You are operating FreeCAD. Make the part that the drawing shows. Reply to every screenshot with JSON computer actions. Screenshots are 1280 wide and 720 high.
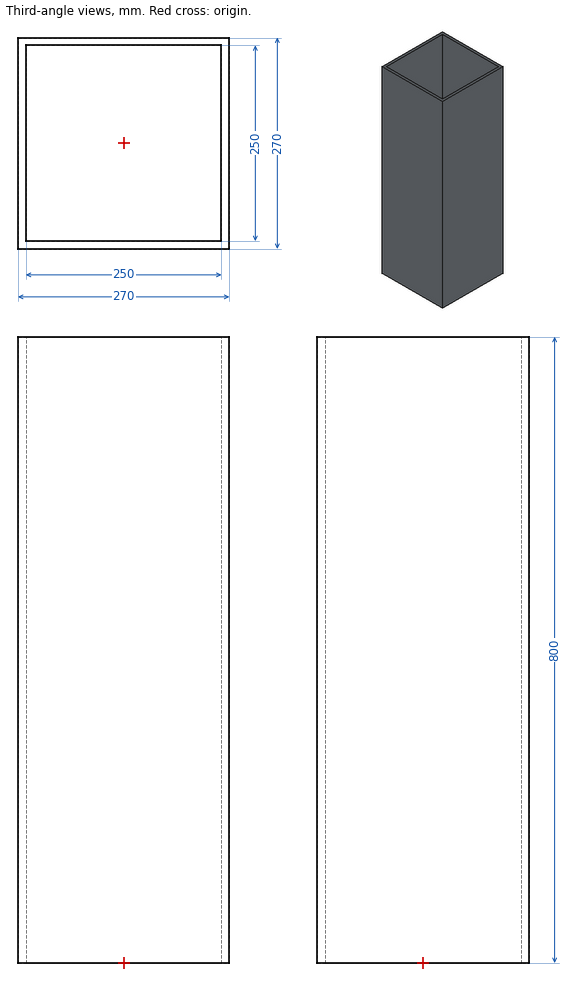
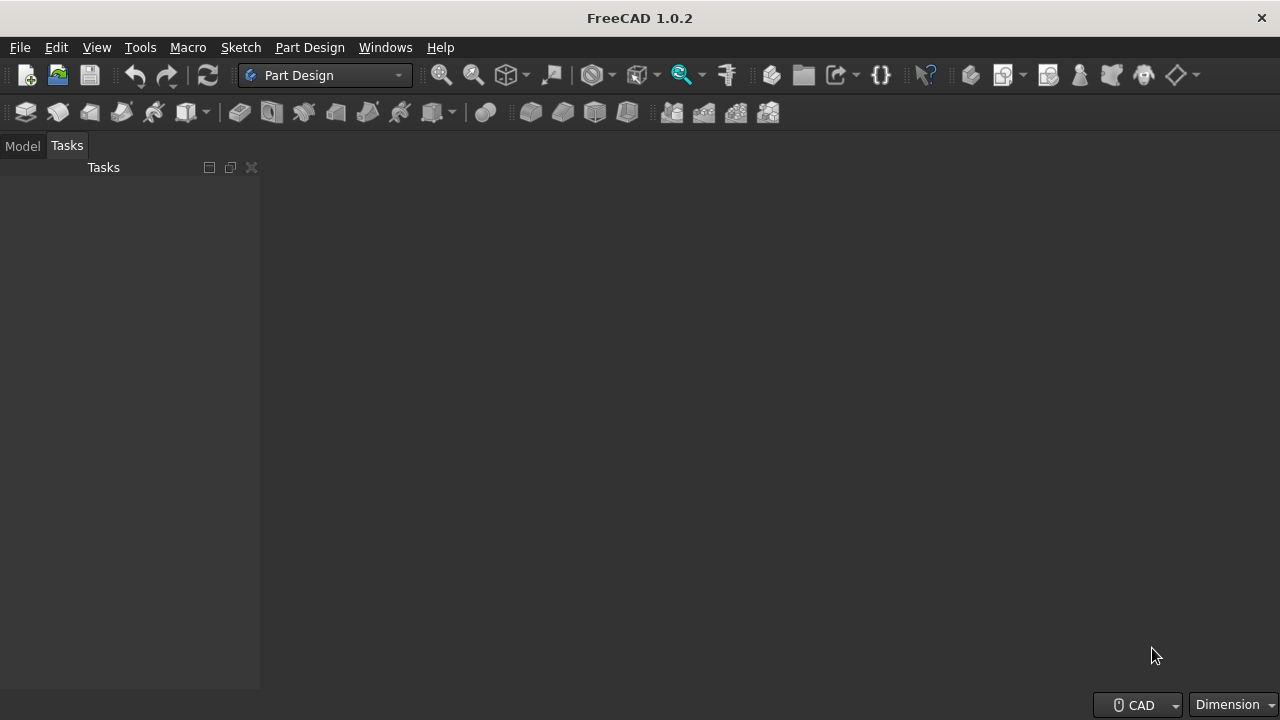
{"action": "left_click", "coordinate": [26, 76]}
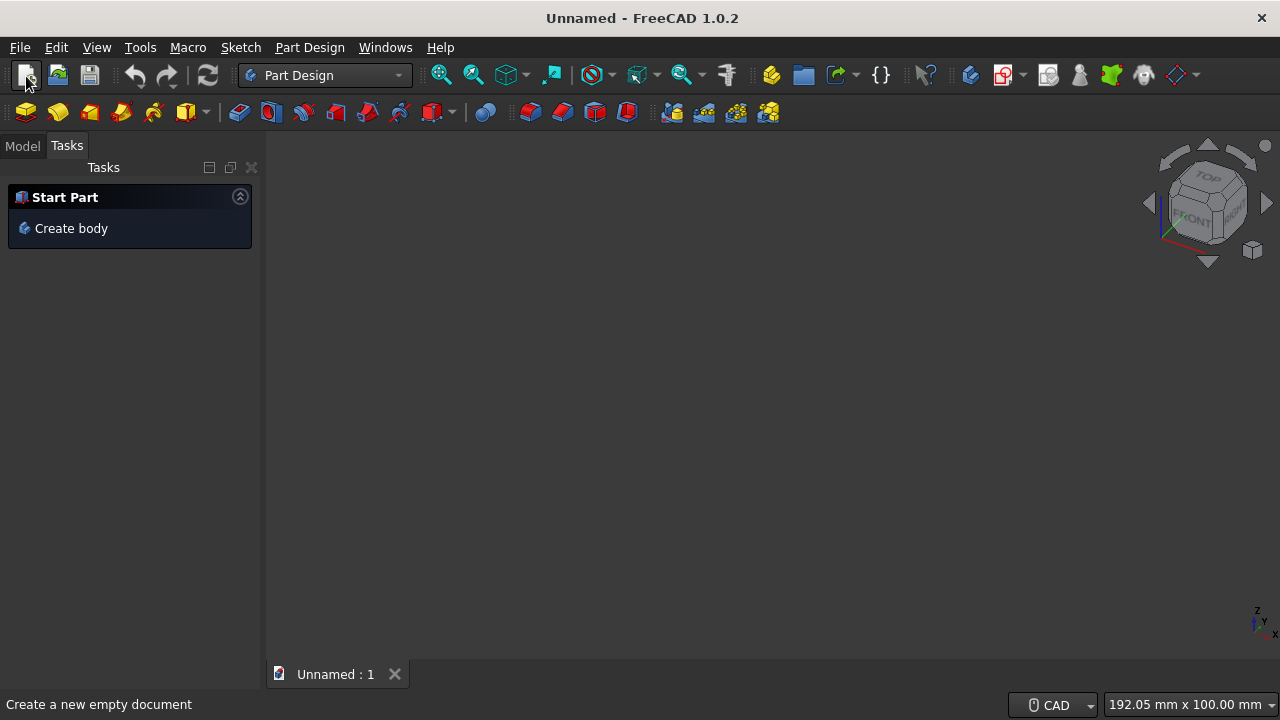
{"action": "left_click", "coordinate": [1004, 76]}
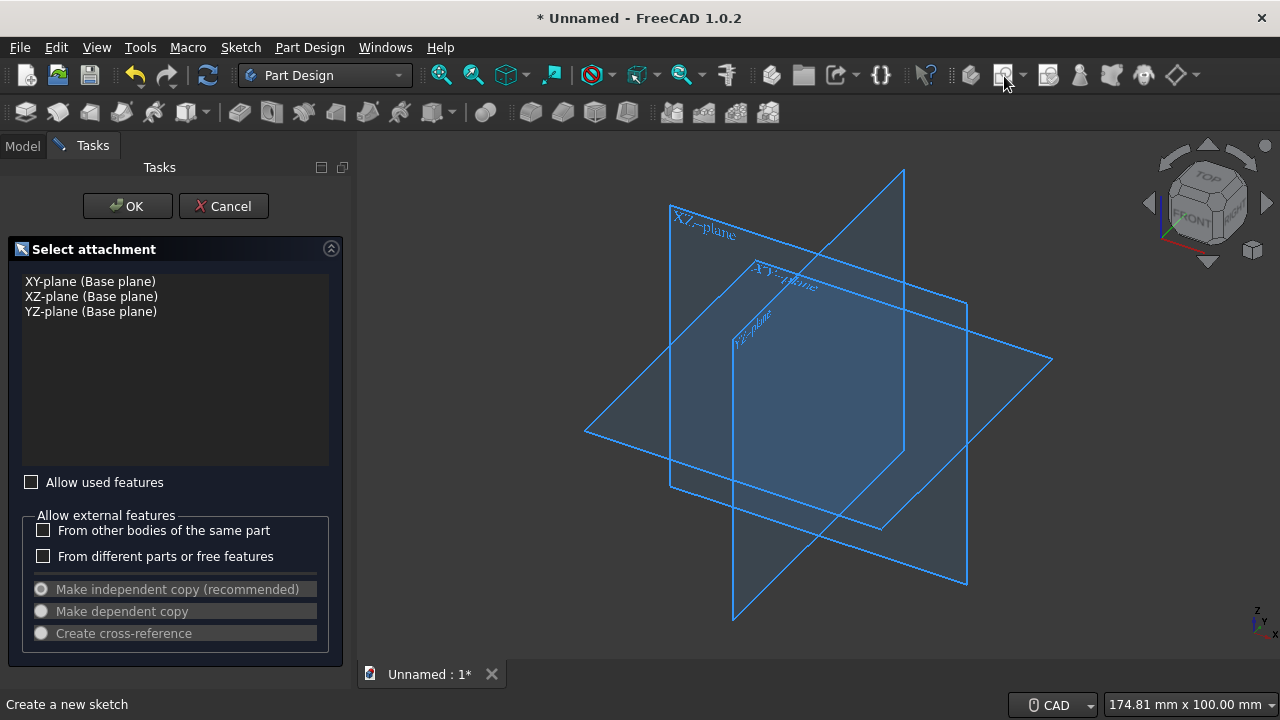
{"action": "left_click", "coordinate": [82, 282]}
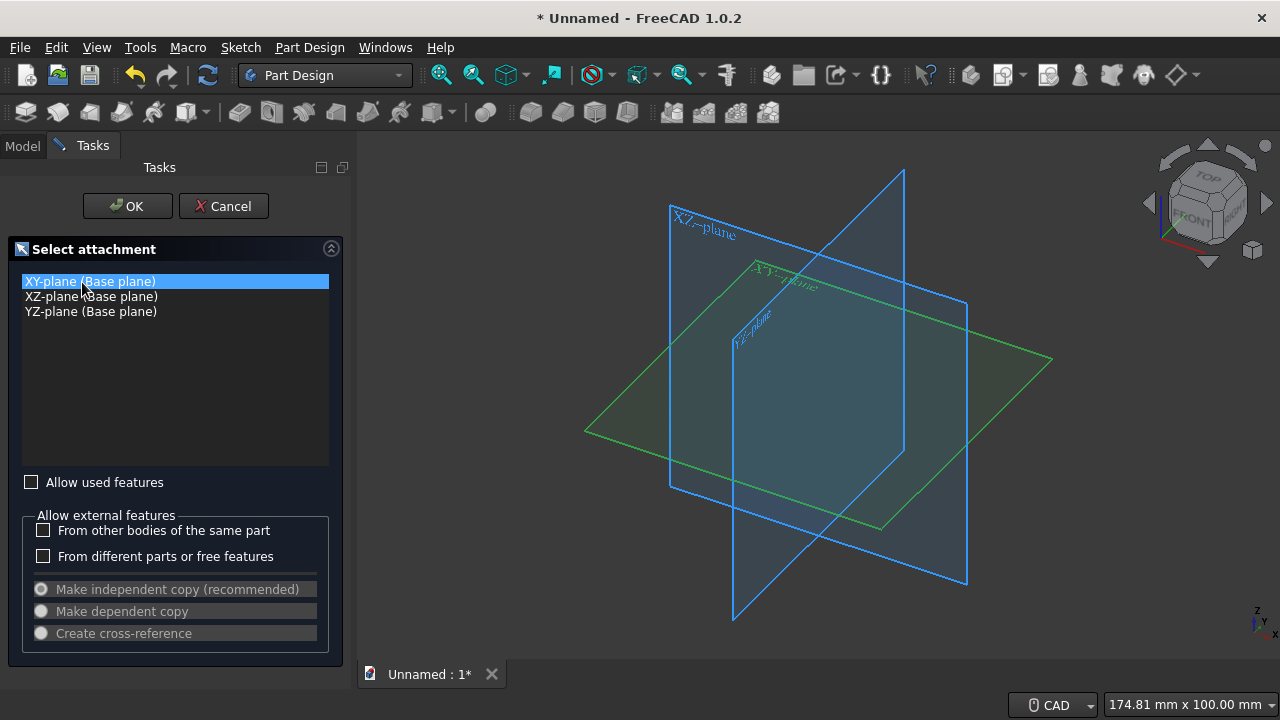
{"action": "left_click", "coordinate": [128, 206]}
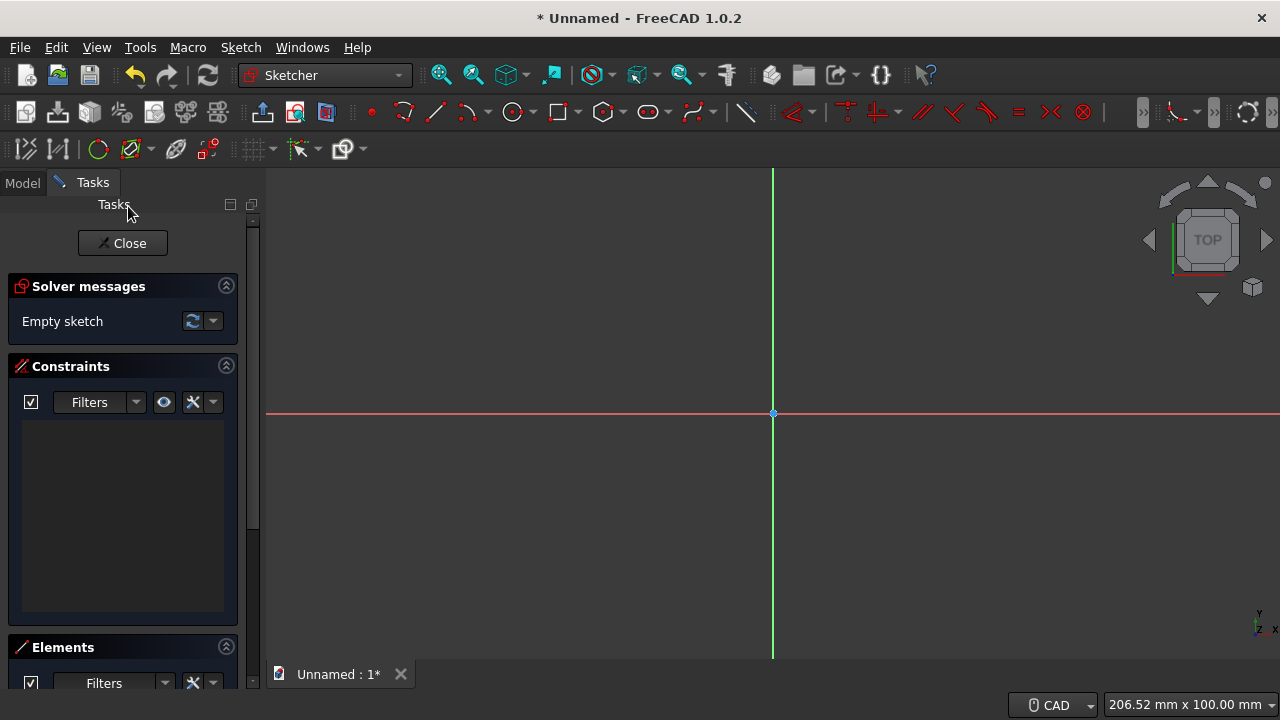
{"action": "scroll", "coordinate": [682, 414], "scroll_direction": "down", "scroll_amount": 7}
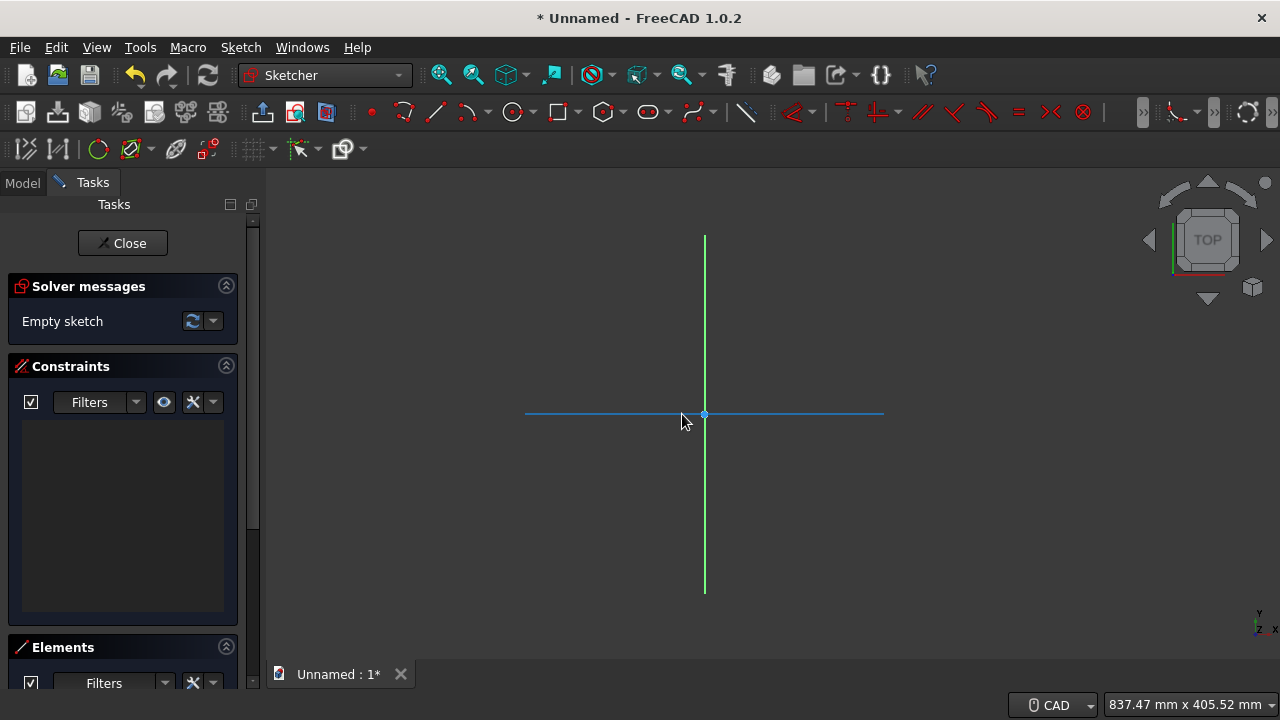
{"action": "key", "text": "g v"}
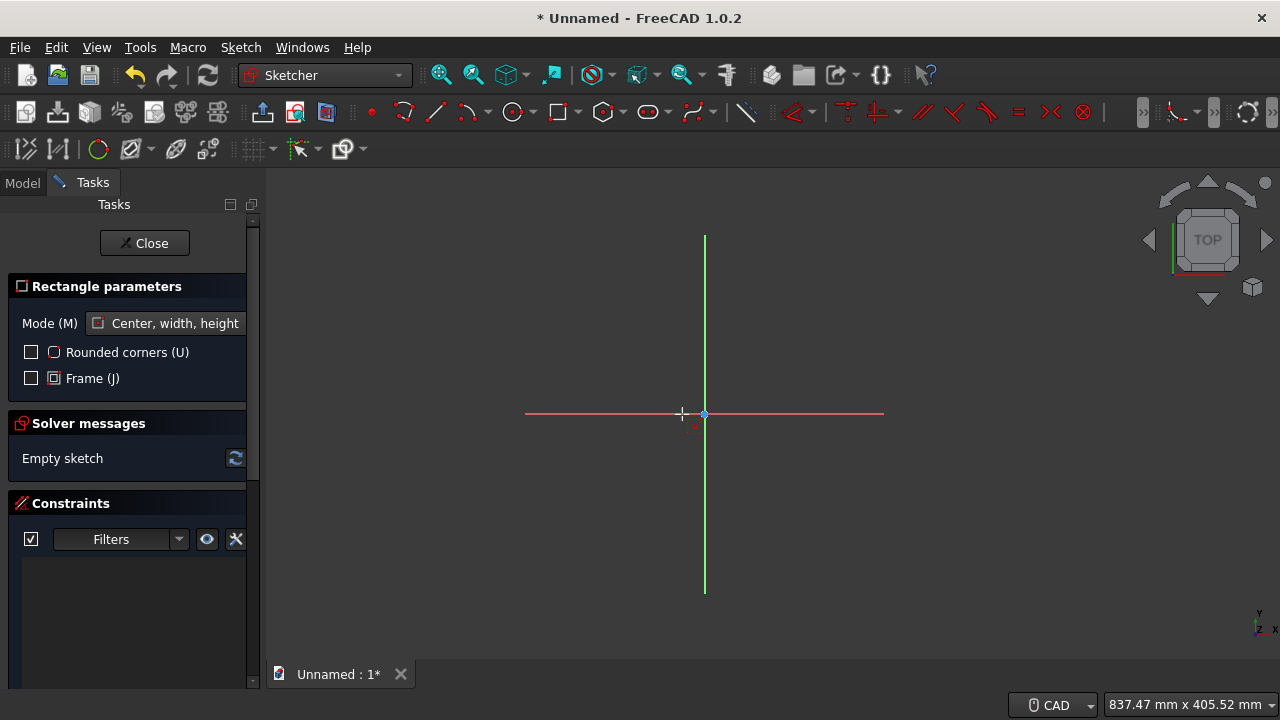
{"action": "left_click", "coordinate": [705, 414]}
{"action": "left_click", "coordinate": [868, 251]}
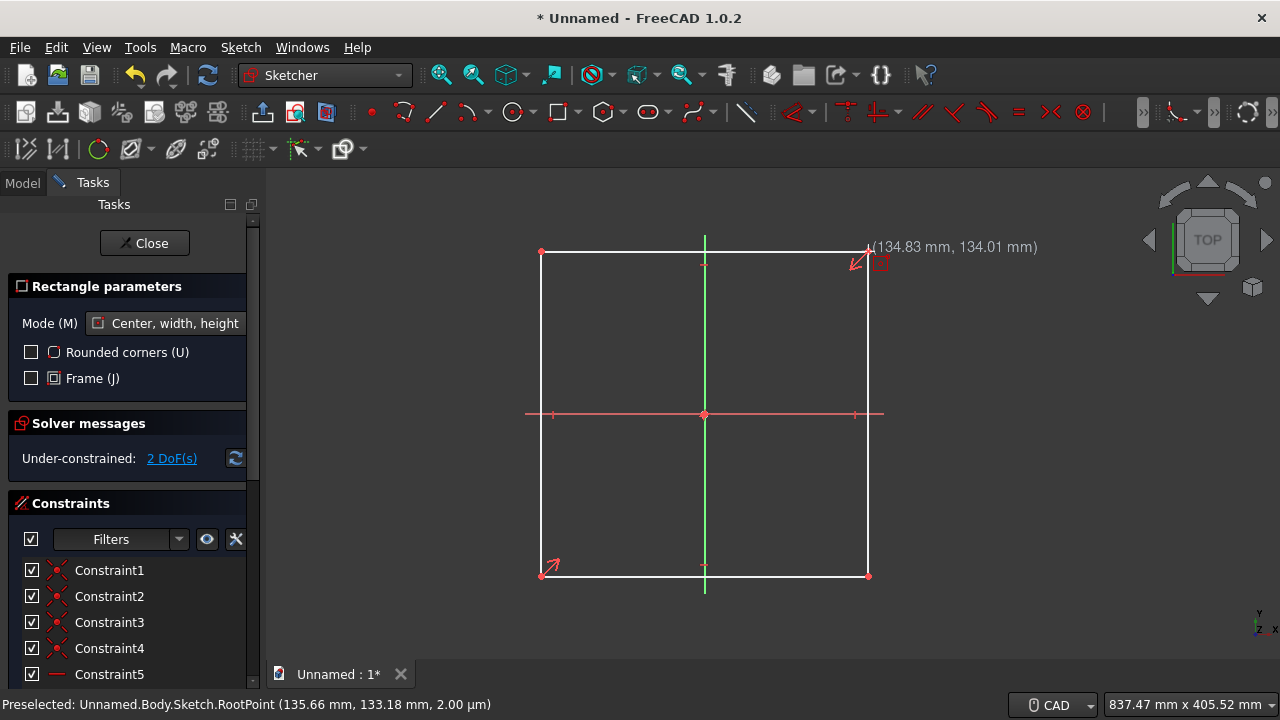
{"action": "left_click", "coordinate": [705, 414]}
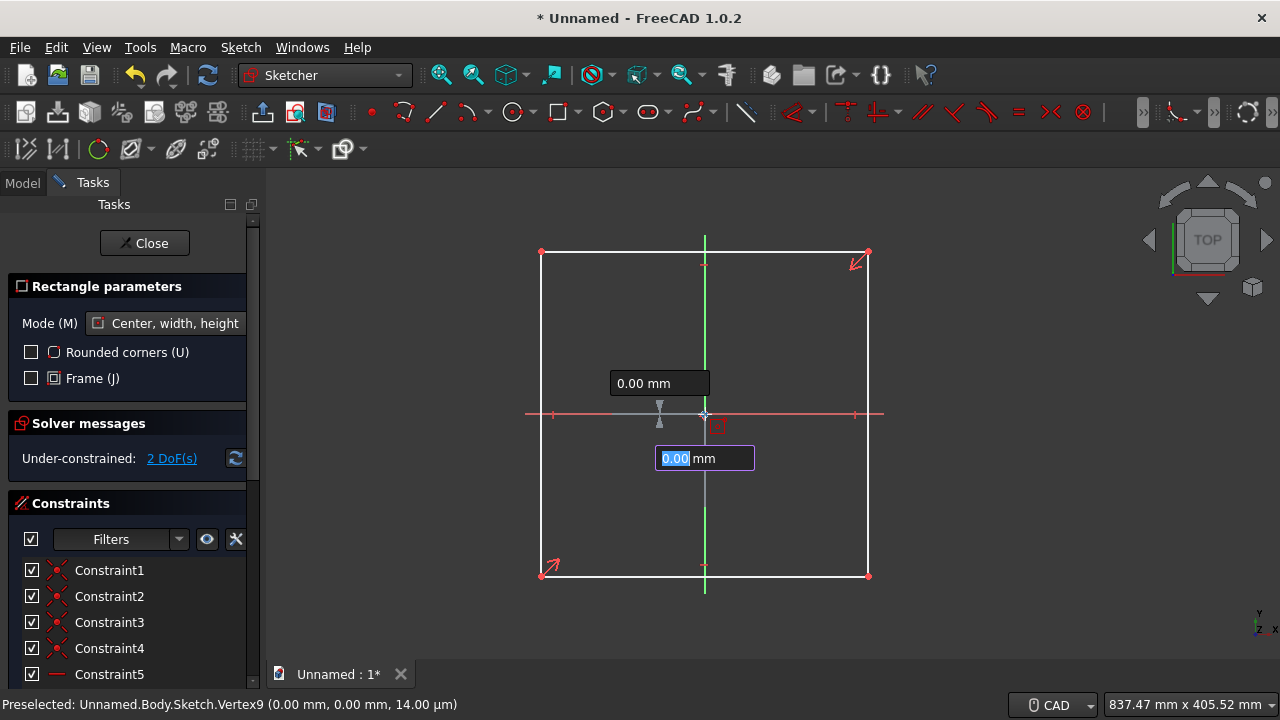
{"action": "scroll", "coordinate": [856, 263], "scroll_direction": "up", "scroll_amount": 2}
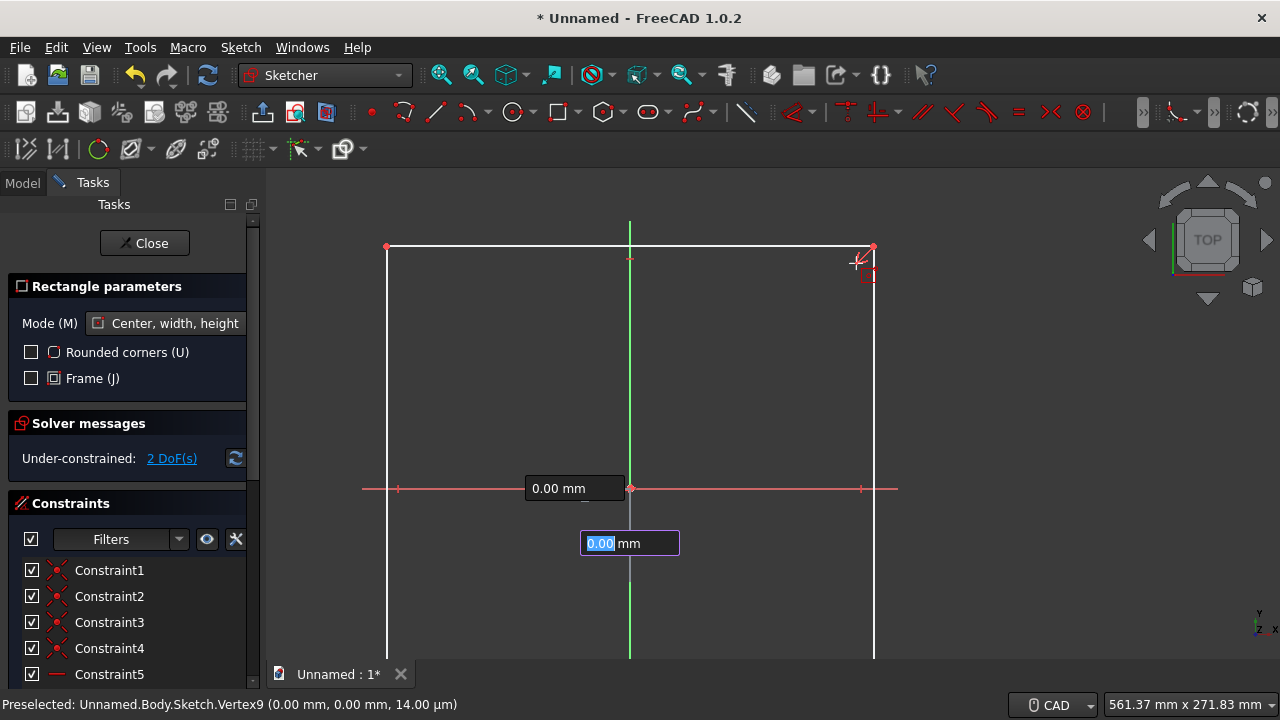
{"action": "left_click", "coordinate": [856, 263]}
{"action": "key", "text": "Escape"}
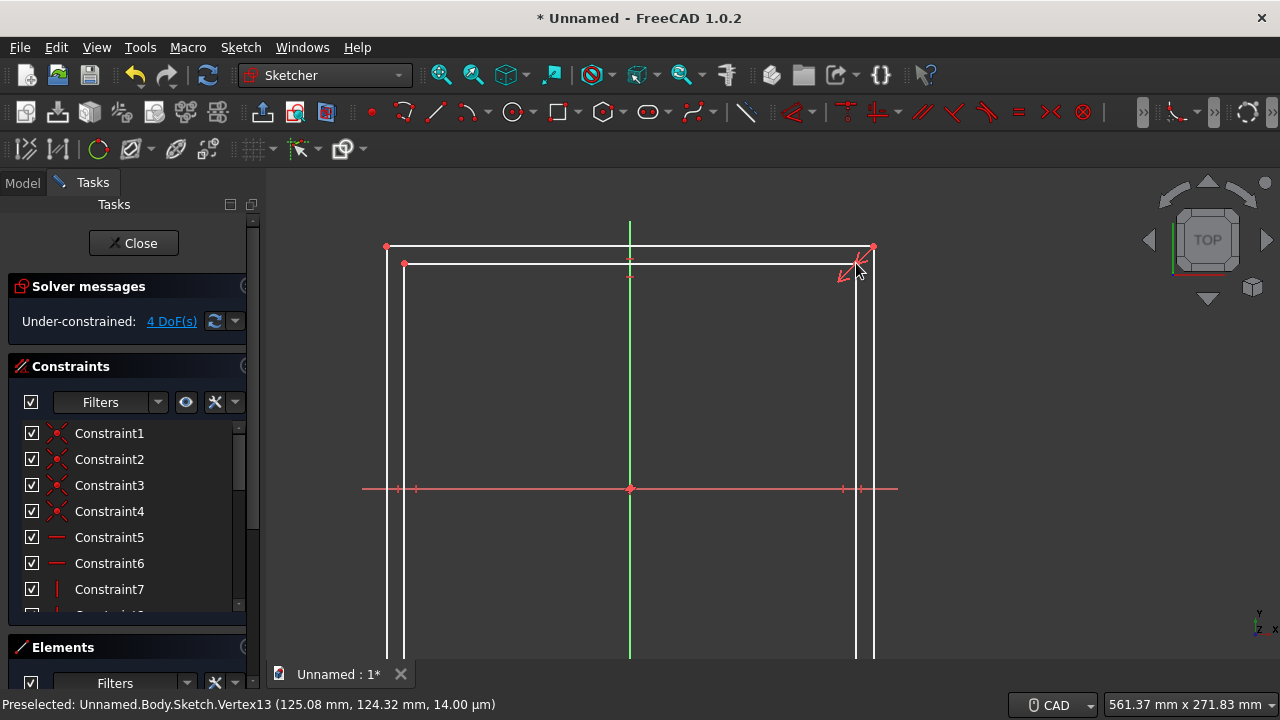
{"action": "scroll", "coordinate": [856, 261], "scroll_direction": "down", "scroll_amount": 2}